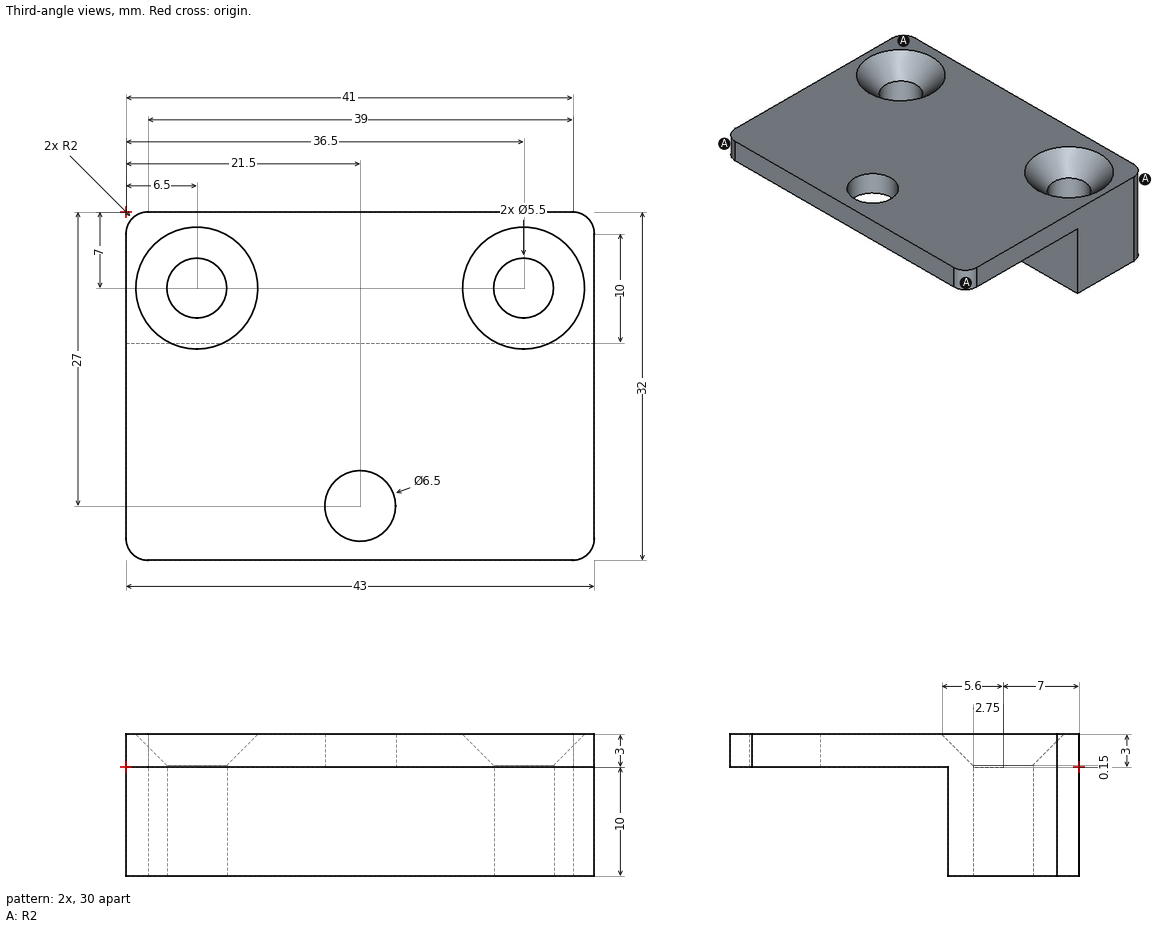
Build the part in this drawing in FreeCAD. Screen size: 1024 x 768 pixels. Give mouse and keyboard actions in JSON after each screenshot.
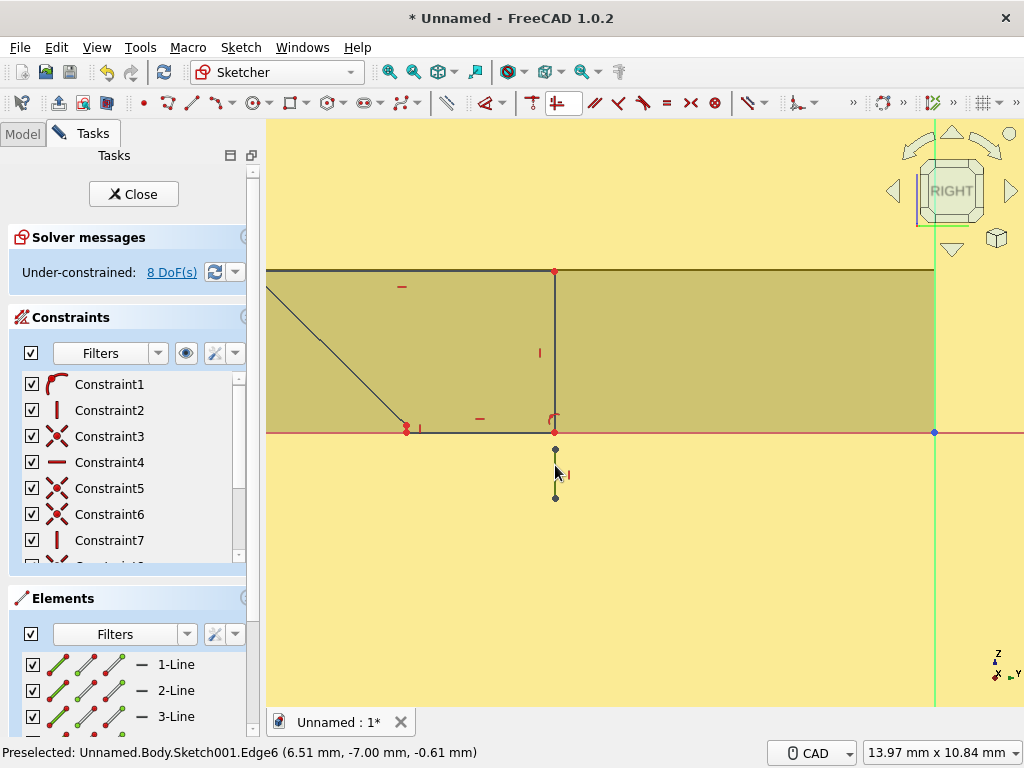
{"action": "key", "text": "g n"}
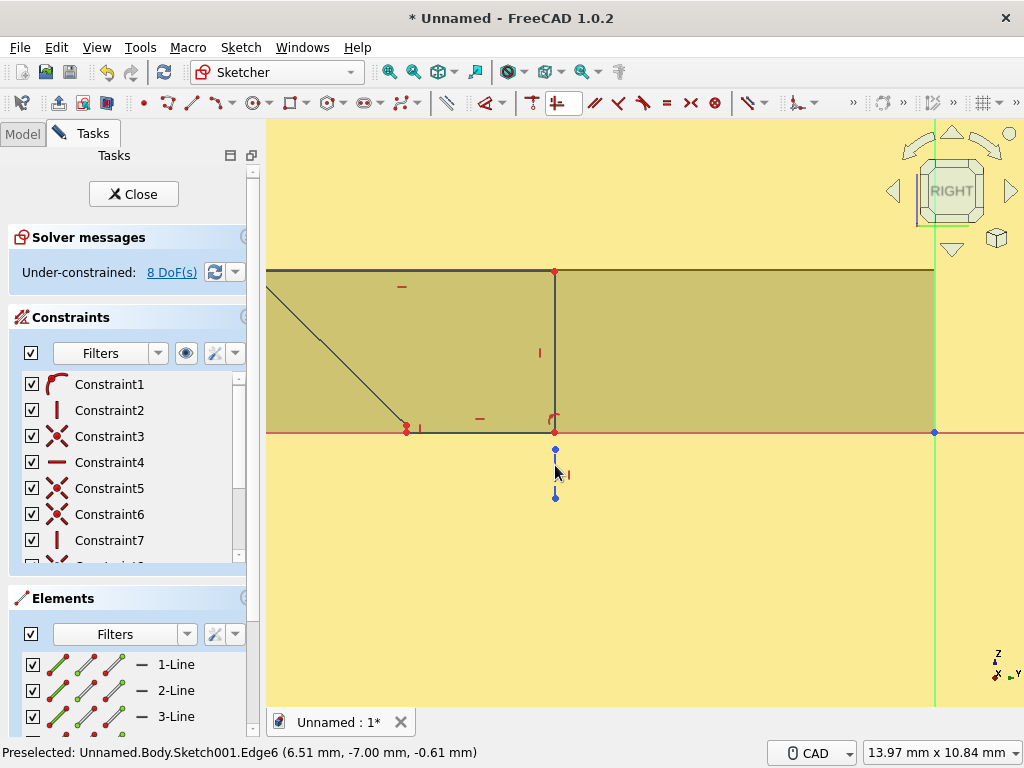
{"action": "key", "text": "d"}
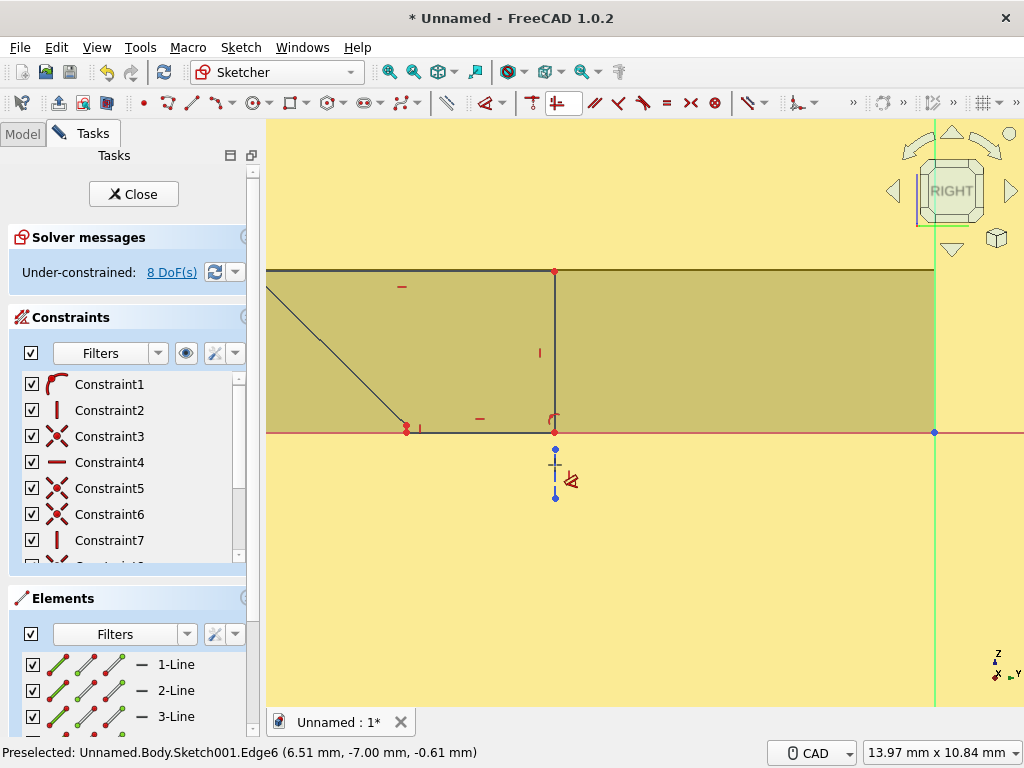
{"action": "left_click", "coordinate": [555, 384]}
{"action": "left_click", "coordinate": [521, 352]}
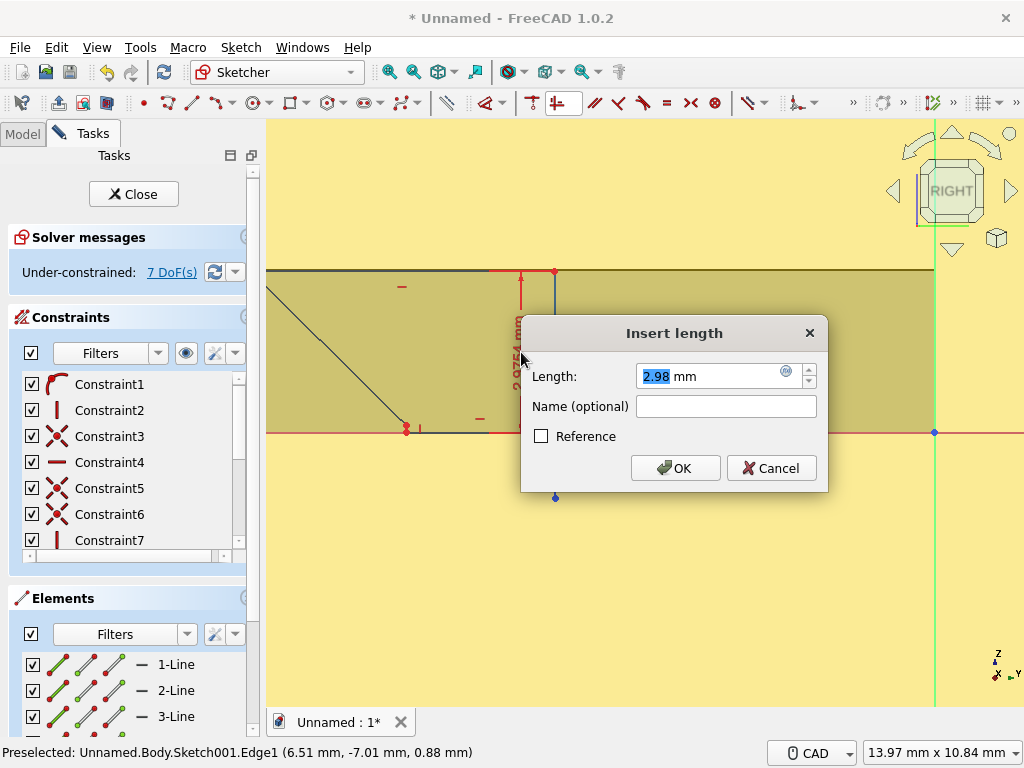
{"action": "type", "text": "3"}
{"action": "key", "text": "Return"}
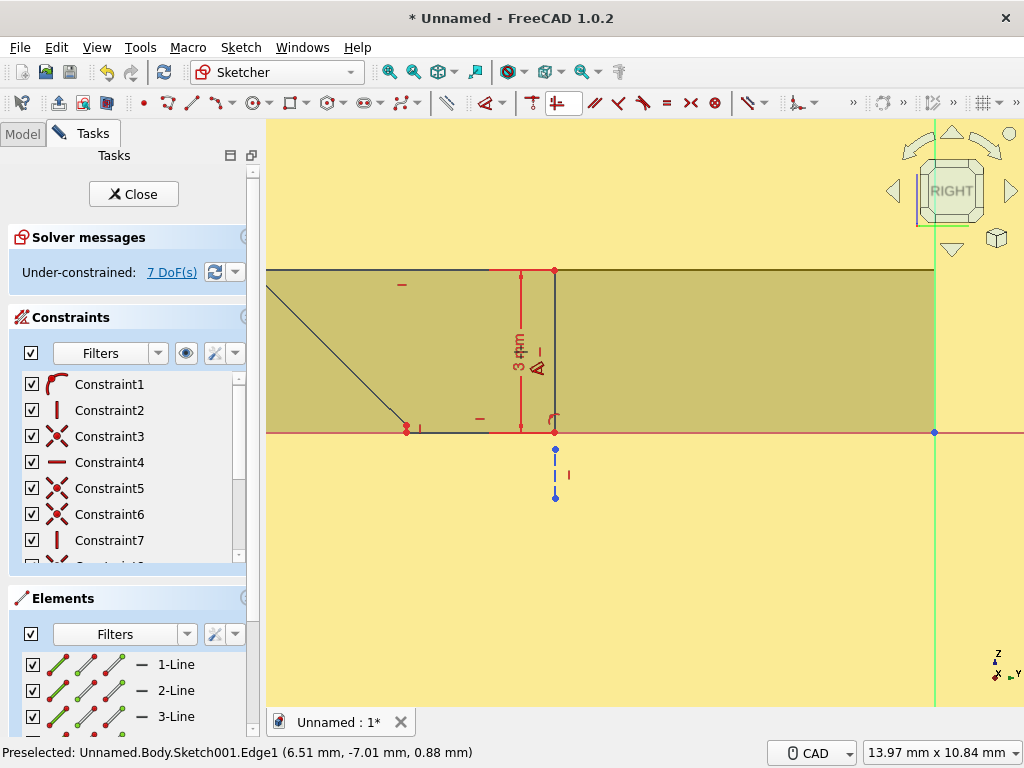
{"action": "left_click", "coordinate": [555, 433]}
{"action": "left_click", "coordinate": [707, 467]}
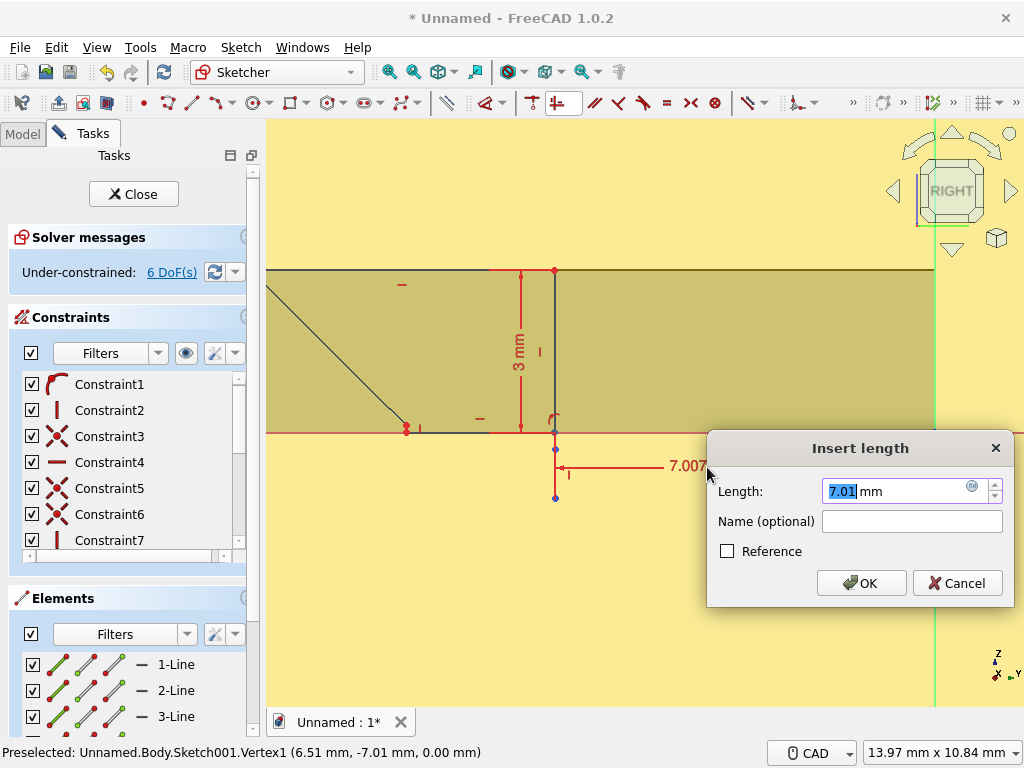
{"action": "type", "text": "7"}
{"action": "key", "text": "Return"}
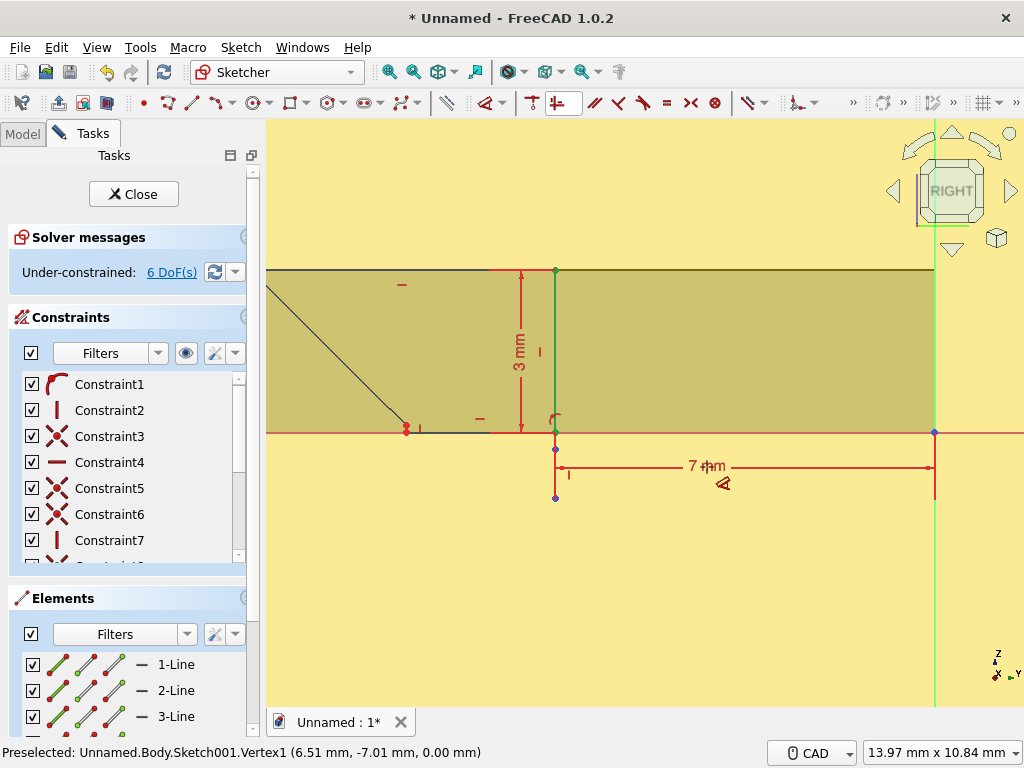
{"action": "left_click", "coordinate": [555, 450]}
{"action": "left_click", "coordinate": [777, 484]}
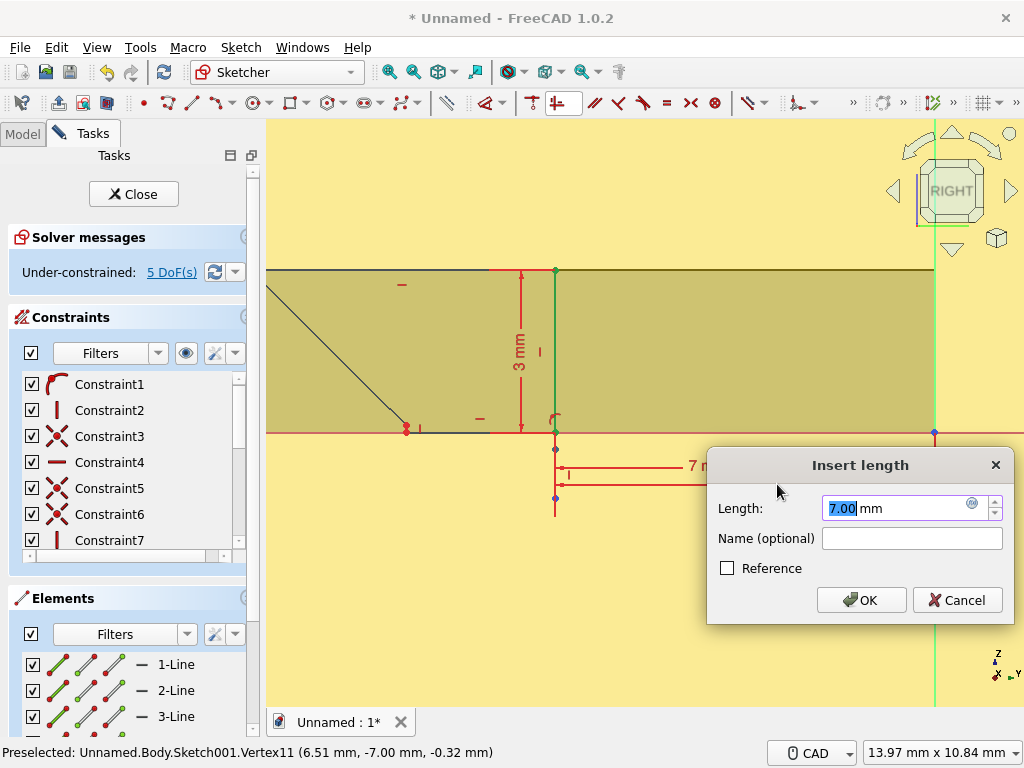
{"action": "type", "text": "7"}
{"action": "key", "text": "Return"}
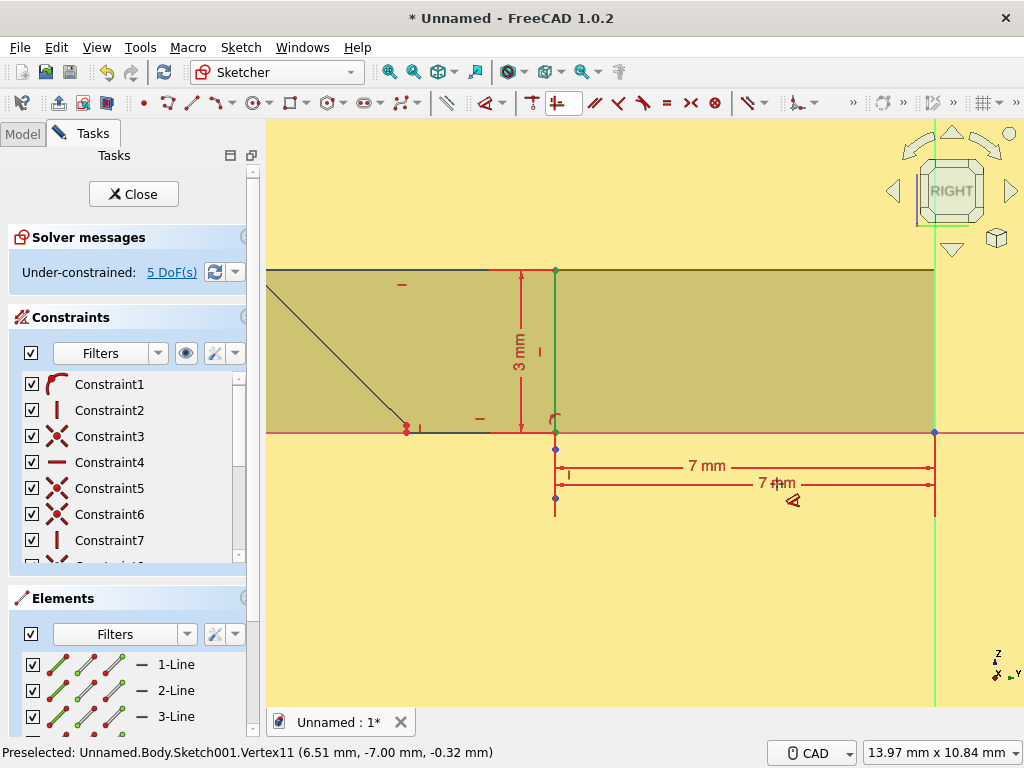
{"action": "left_click", "coordinate": [464, 270]}
{"action": "left_click", "coordinate": [425, 236]}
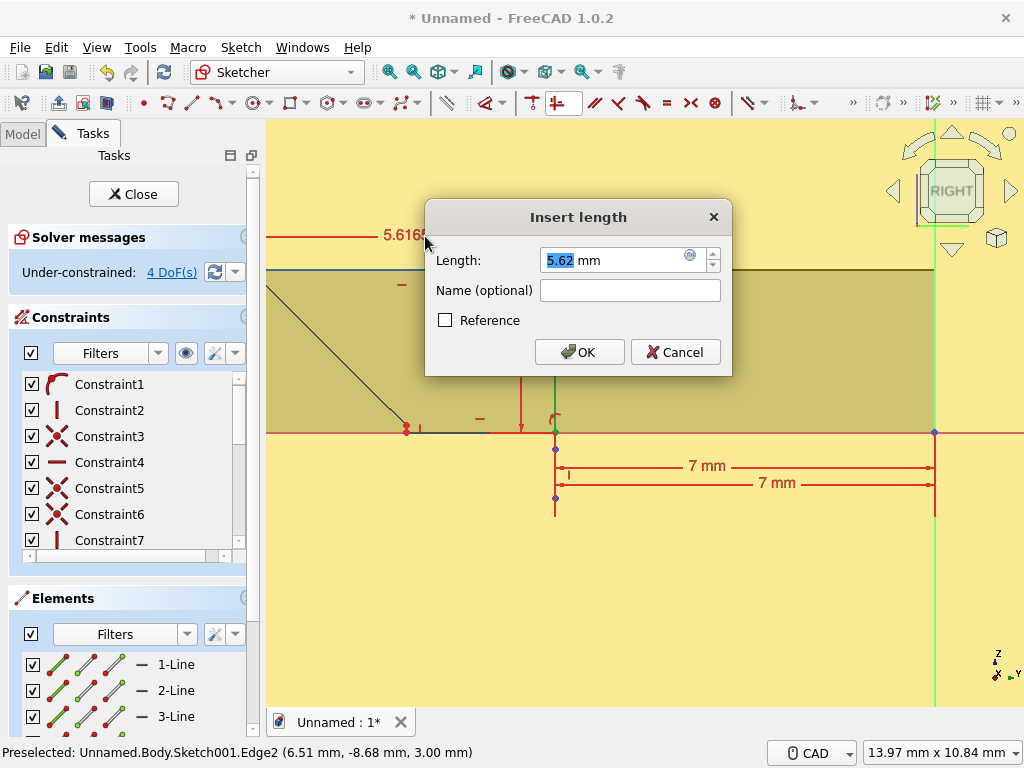
{"action": "type", "text": "5.6"}
{"action": "key", "text": "Return"}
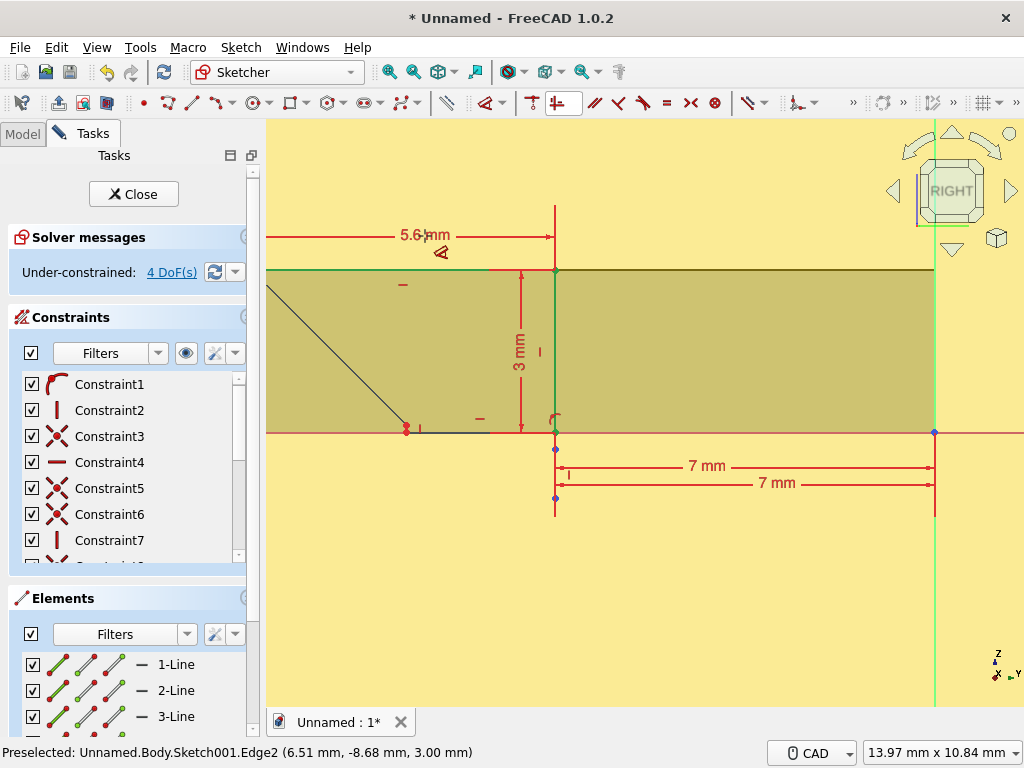
{"action": "scroll", "coordinate": [406, 429], "scroll_direction": "up", "scroll_amount": 8}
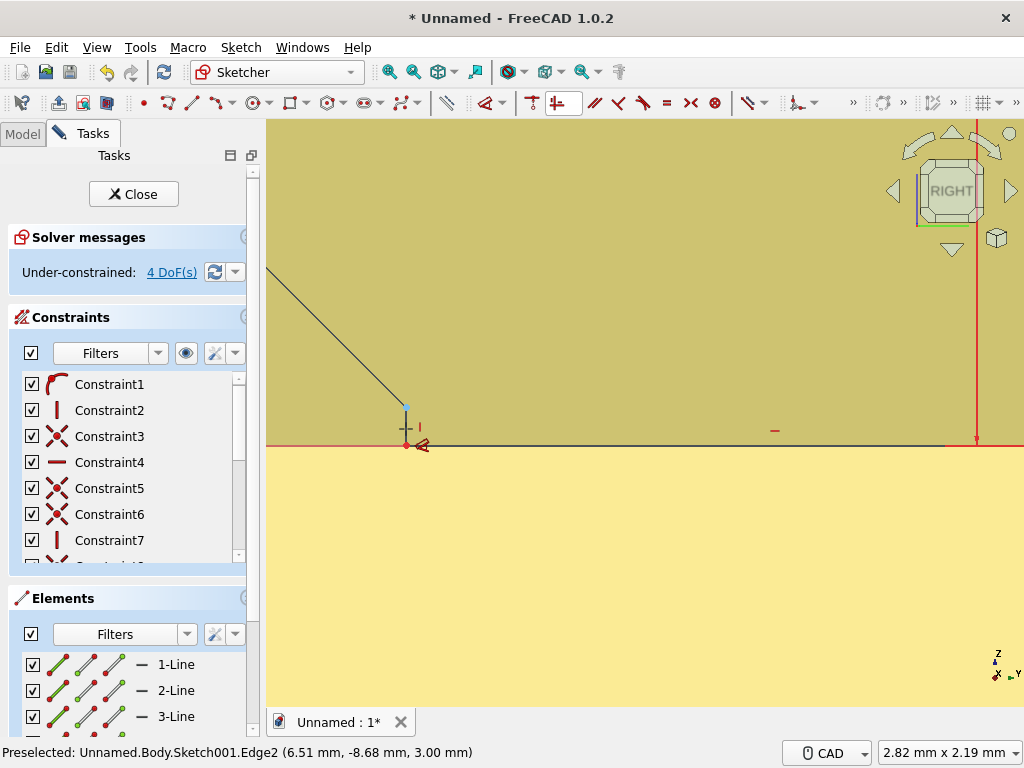
{"action": "left_click", "coordinate": [406, 427]}
{"action": "left_click", "coordinate": [372, 427]}